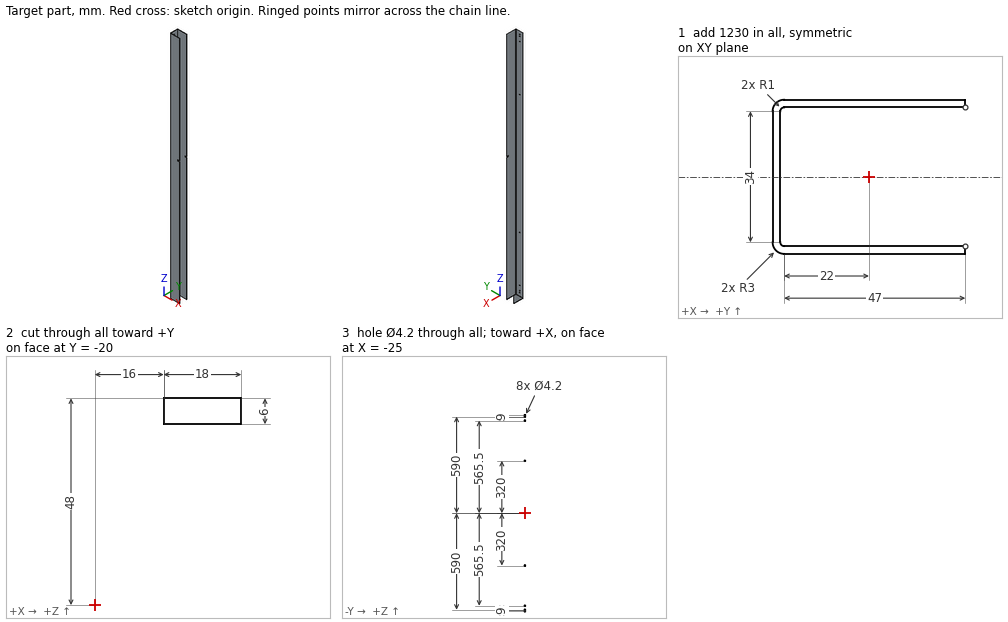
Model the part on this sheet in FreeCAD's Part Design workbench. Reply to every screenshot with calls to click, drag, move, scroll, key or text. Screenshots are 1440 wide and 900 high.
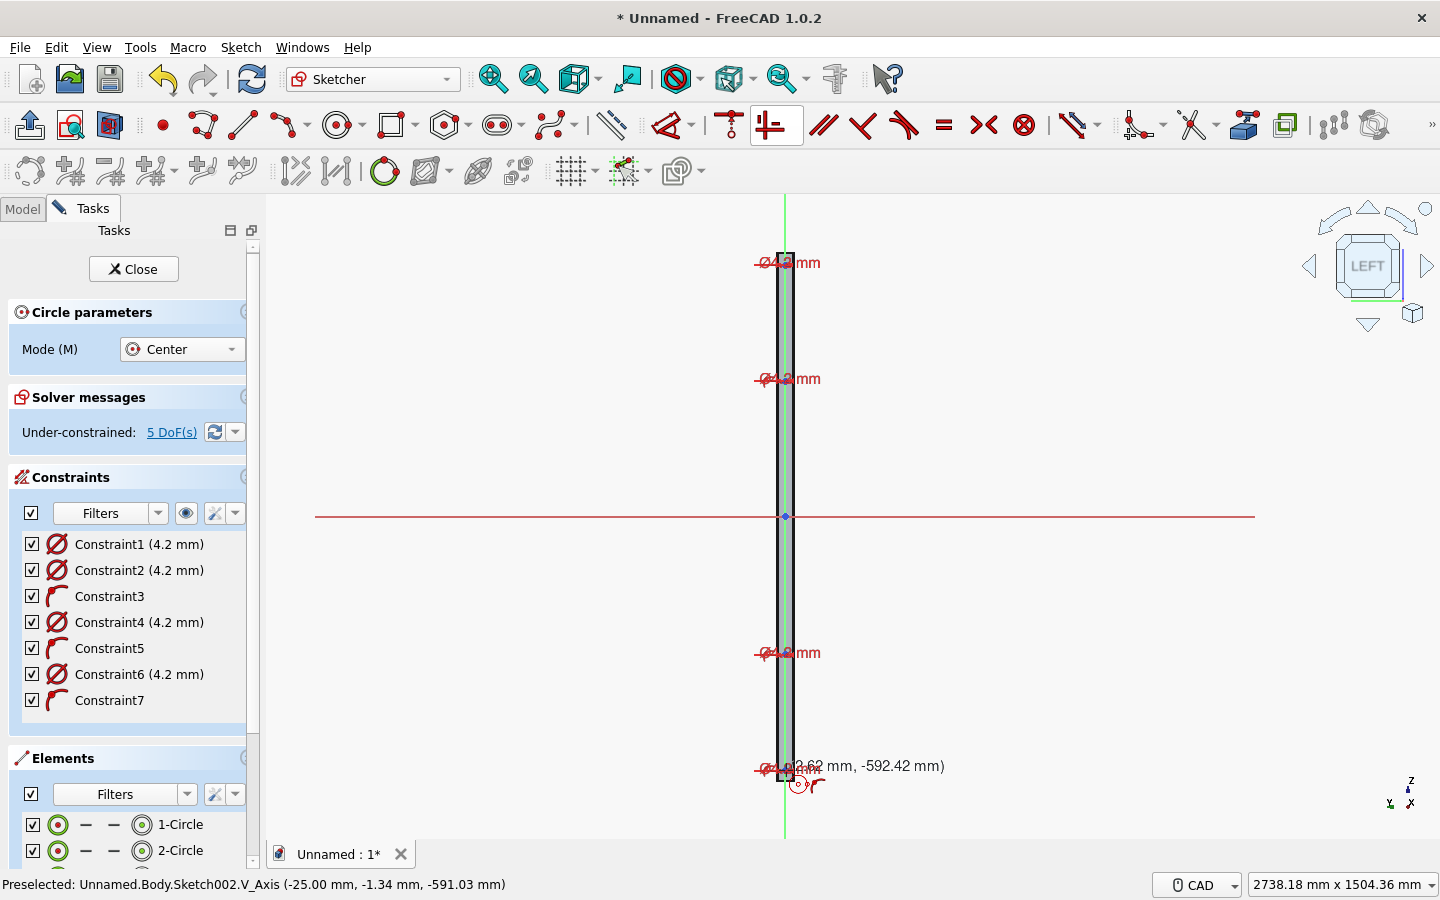
scroll(785, 274, up, 17)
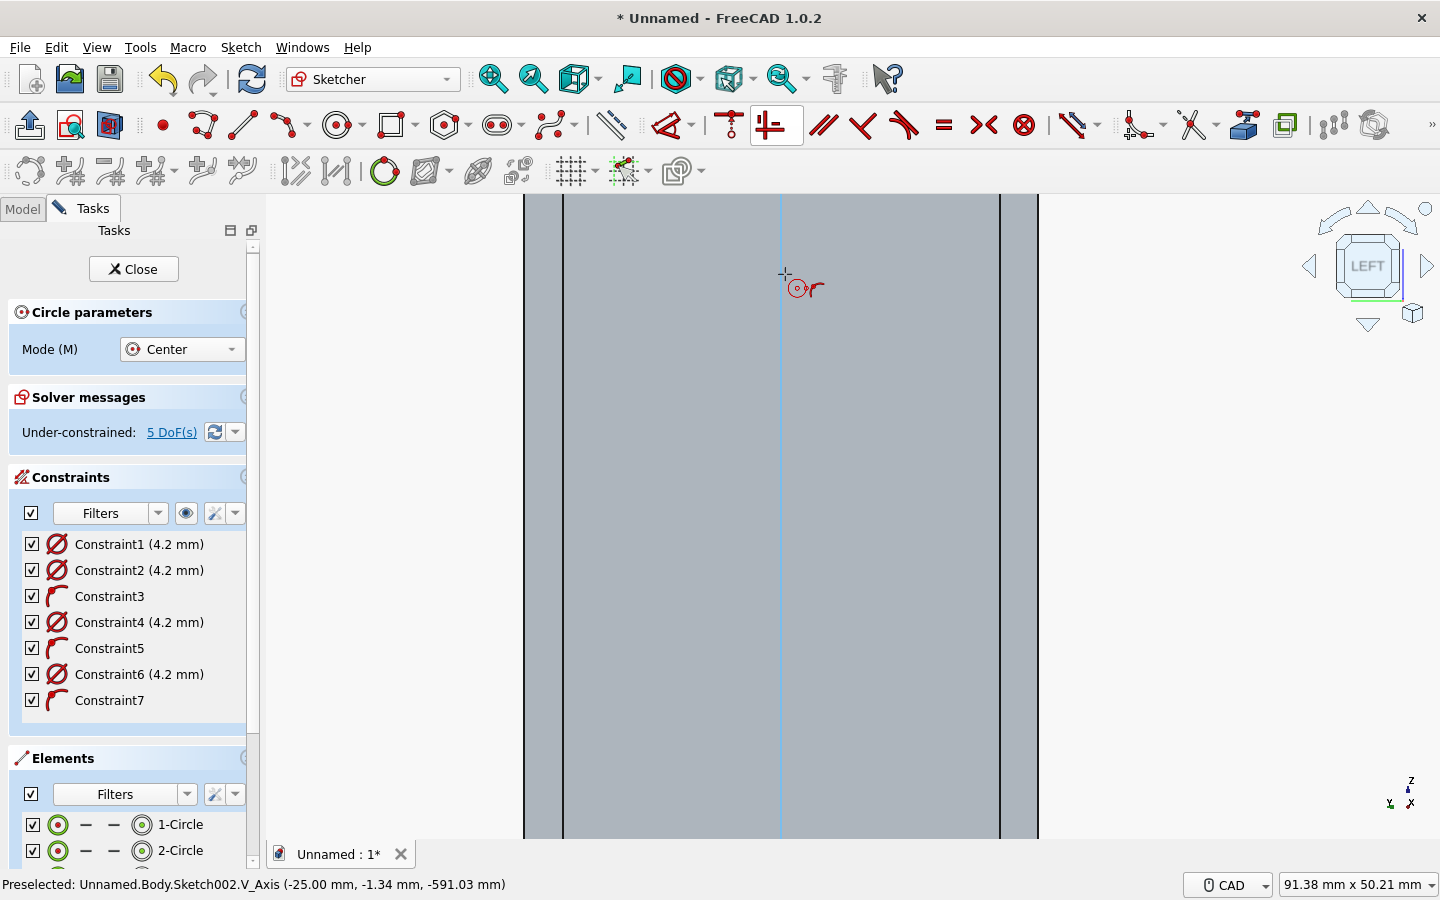
scroll(785, 274, down, 17)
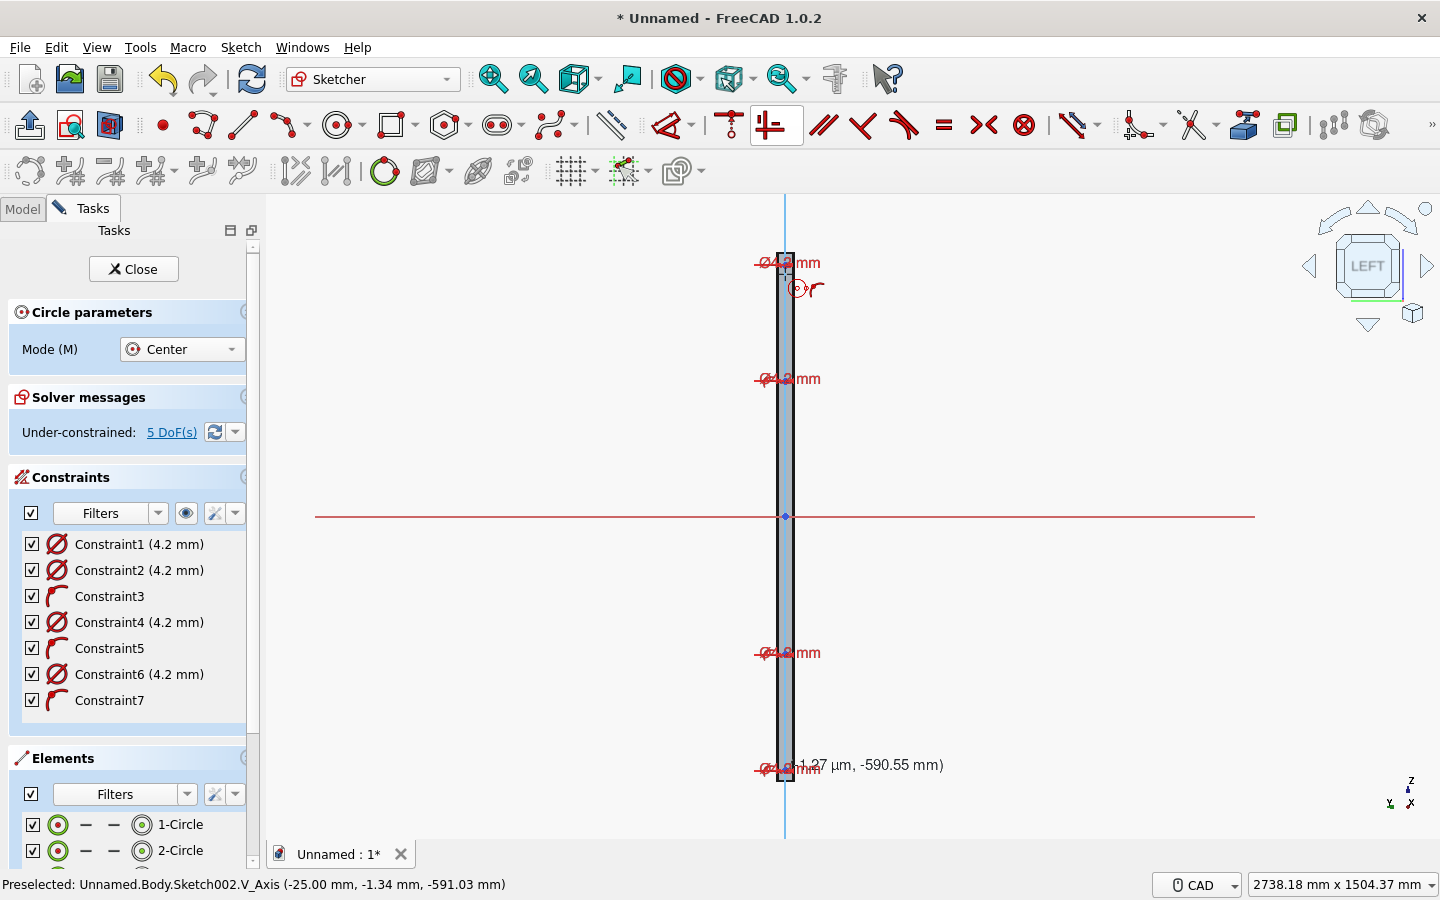
scroll(785, 274, up, 3)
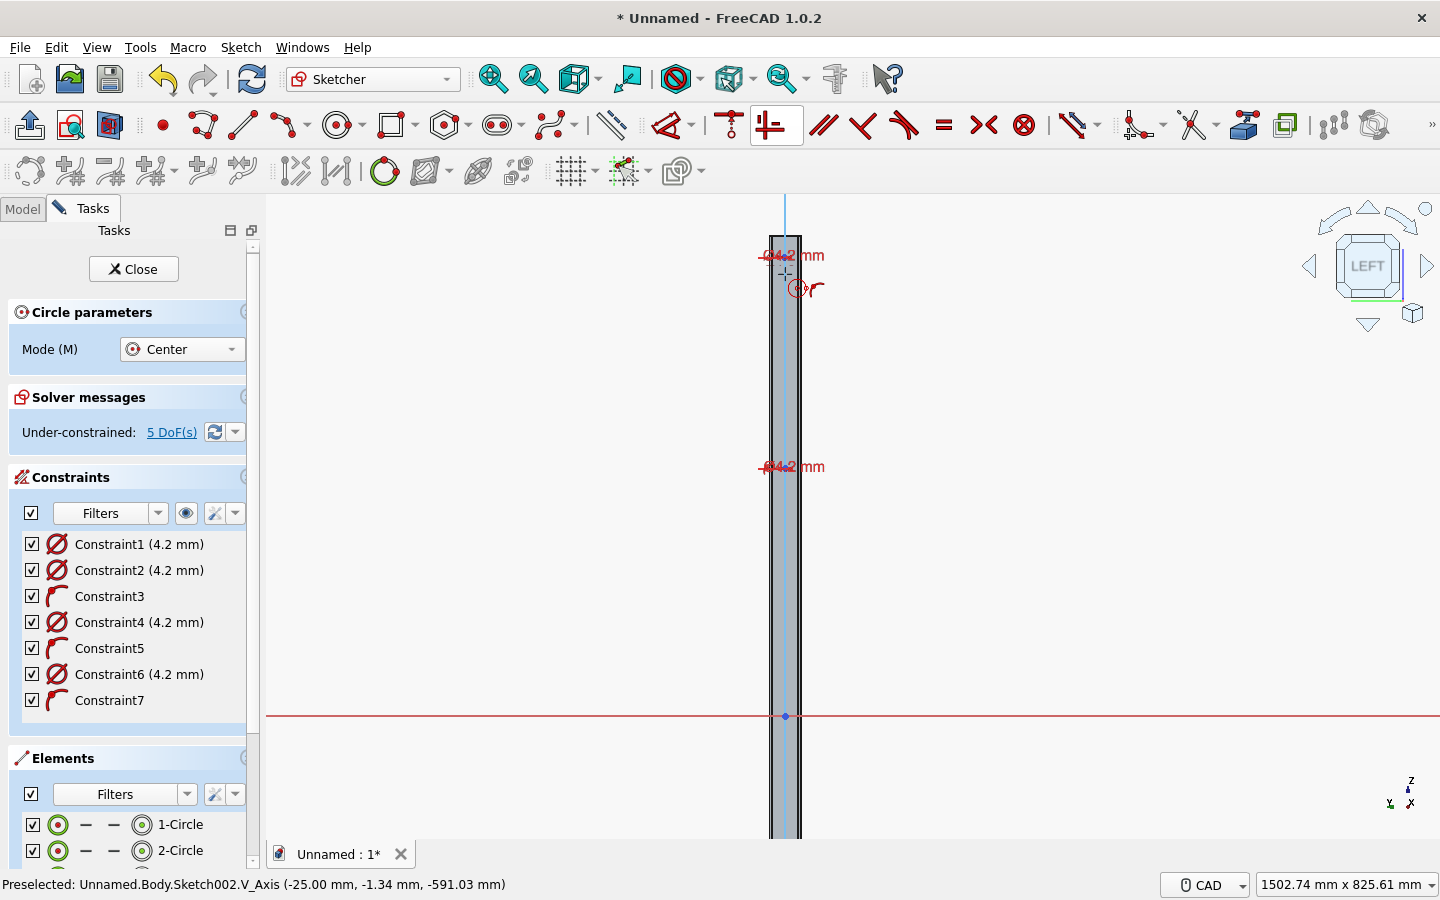
click(785, 275)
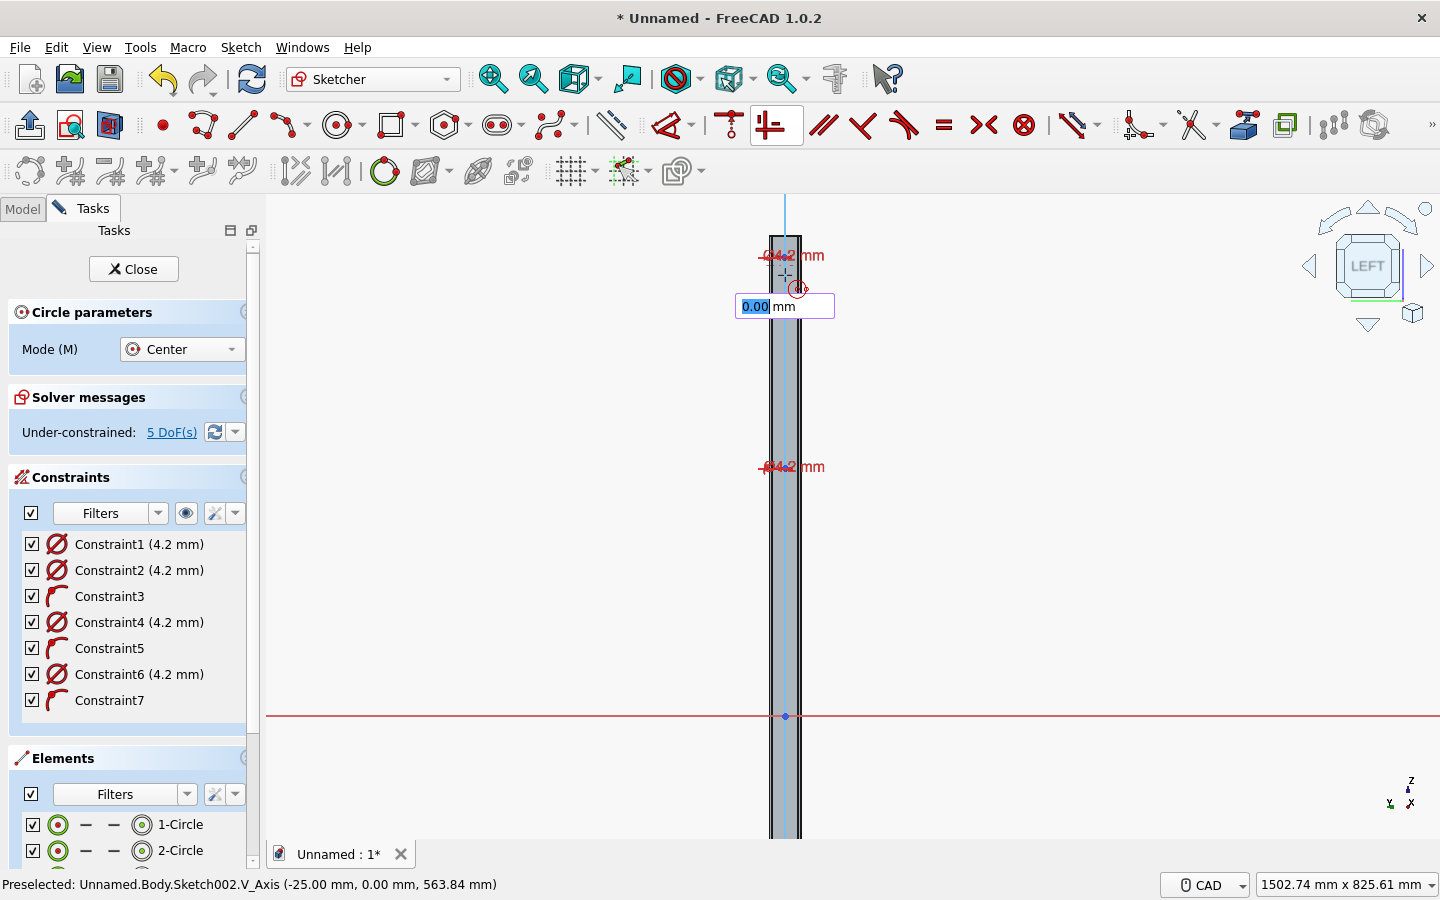
scroll(787, 274, up, 12)
move(779, 274)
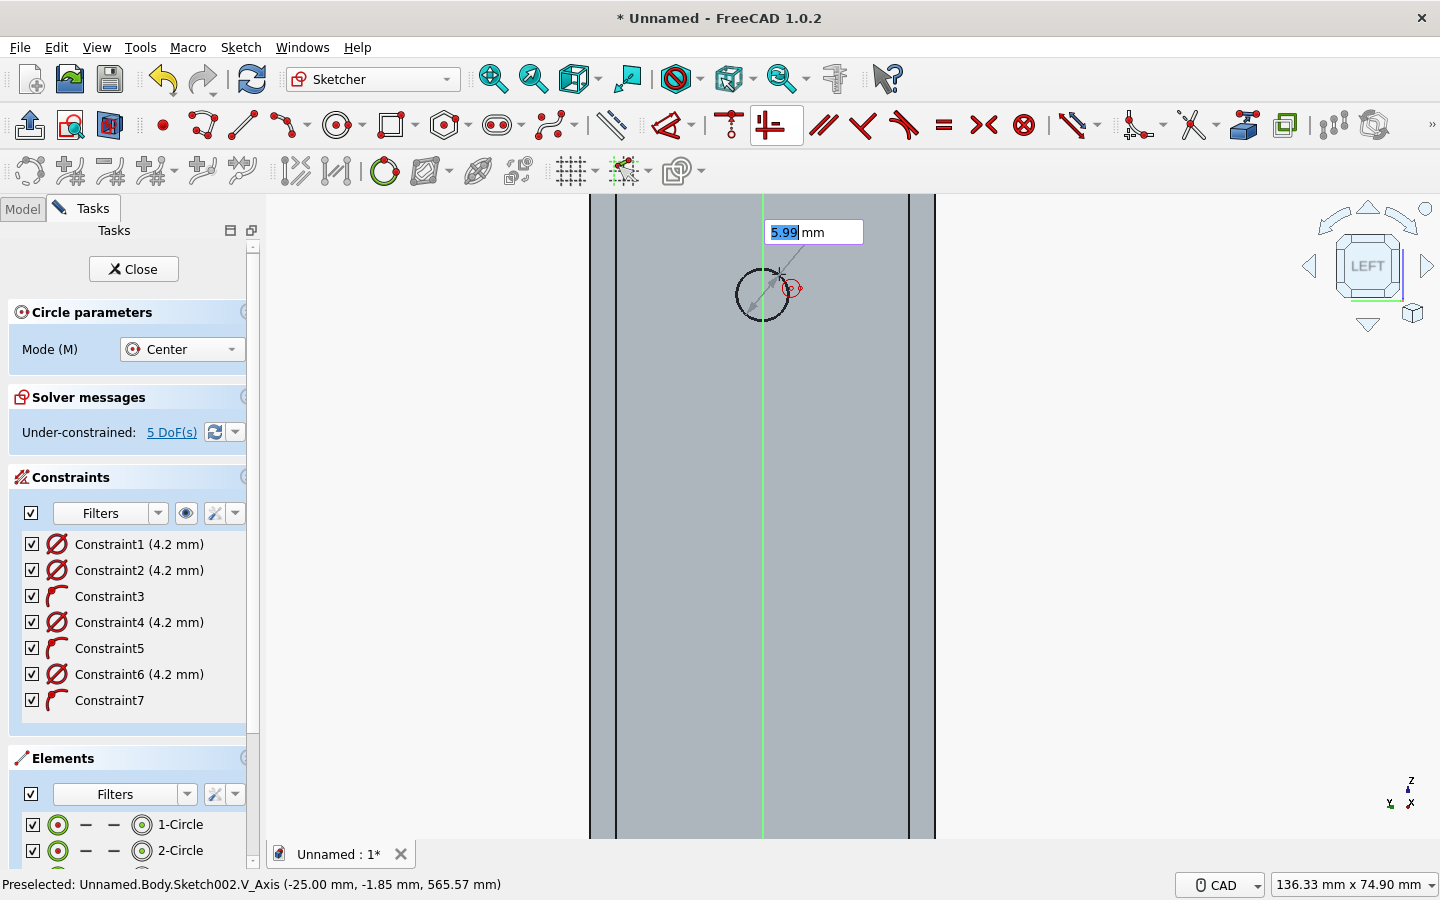
text(4.2)
key(Return)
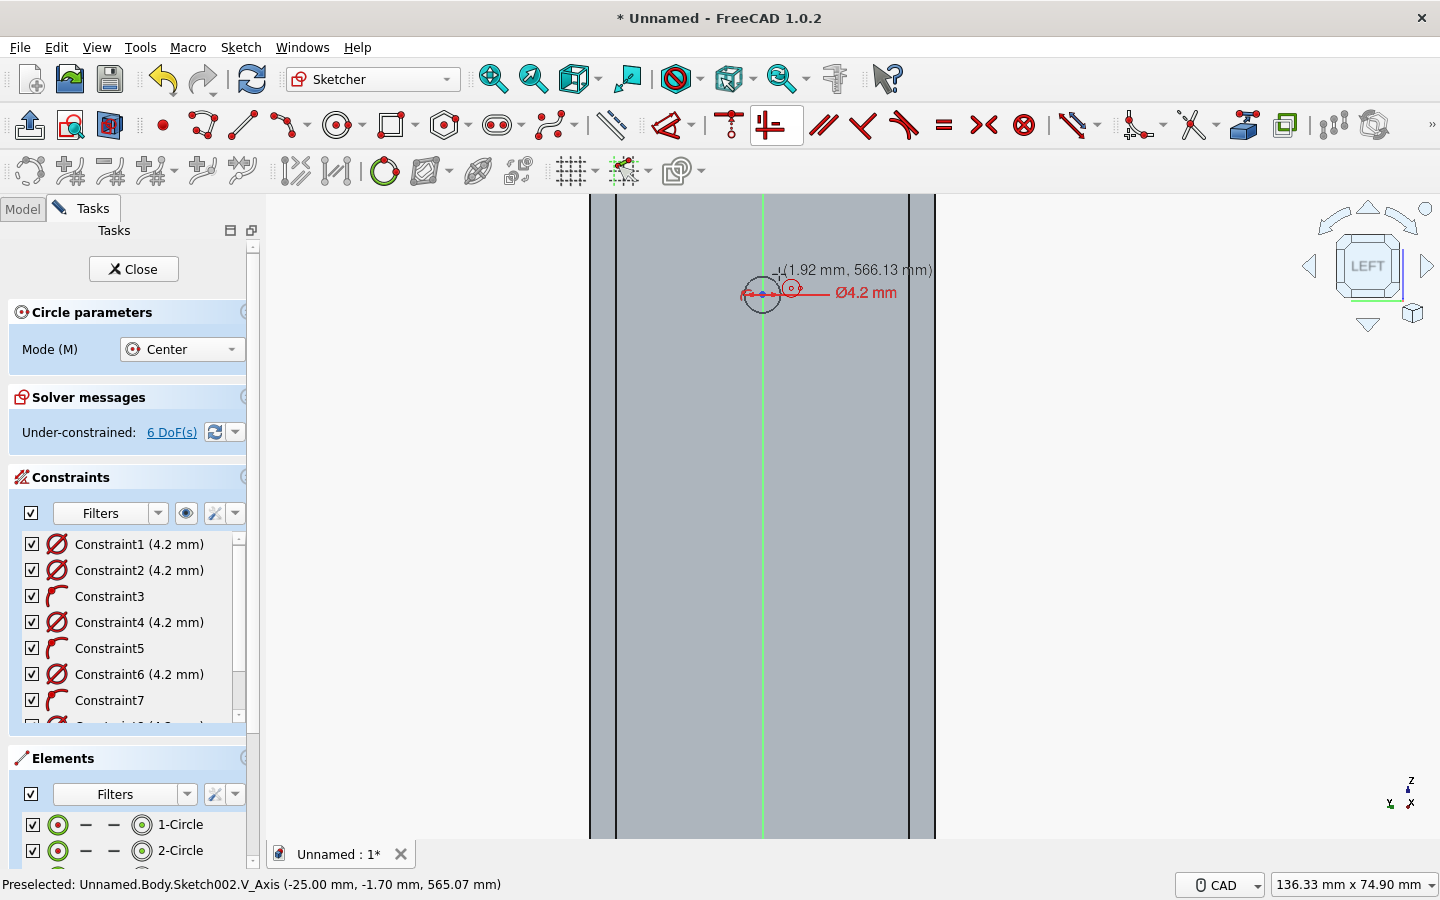
scroll(786, 274, down, 15)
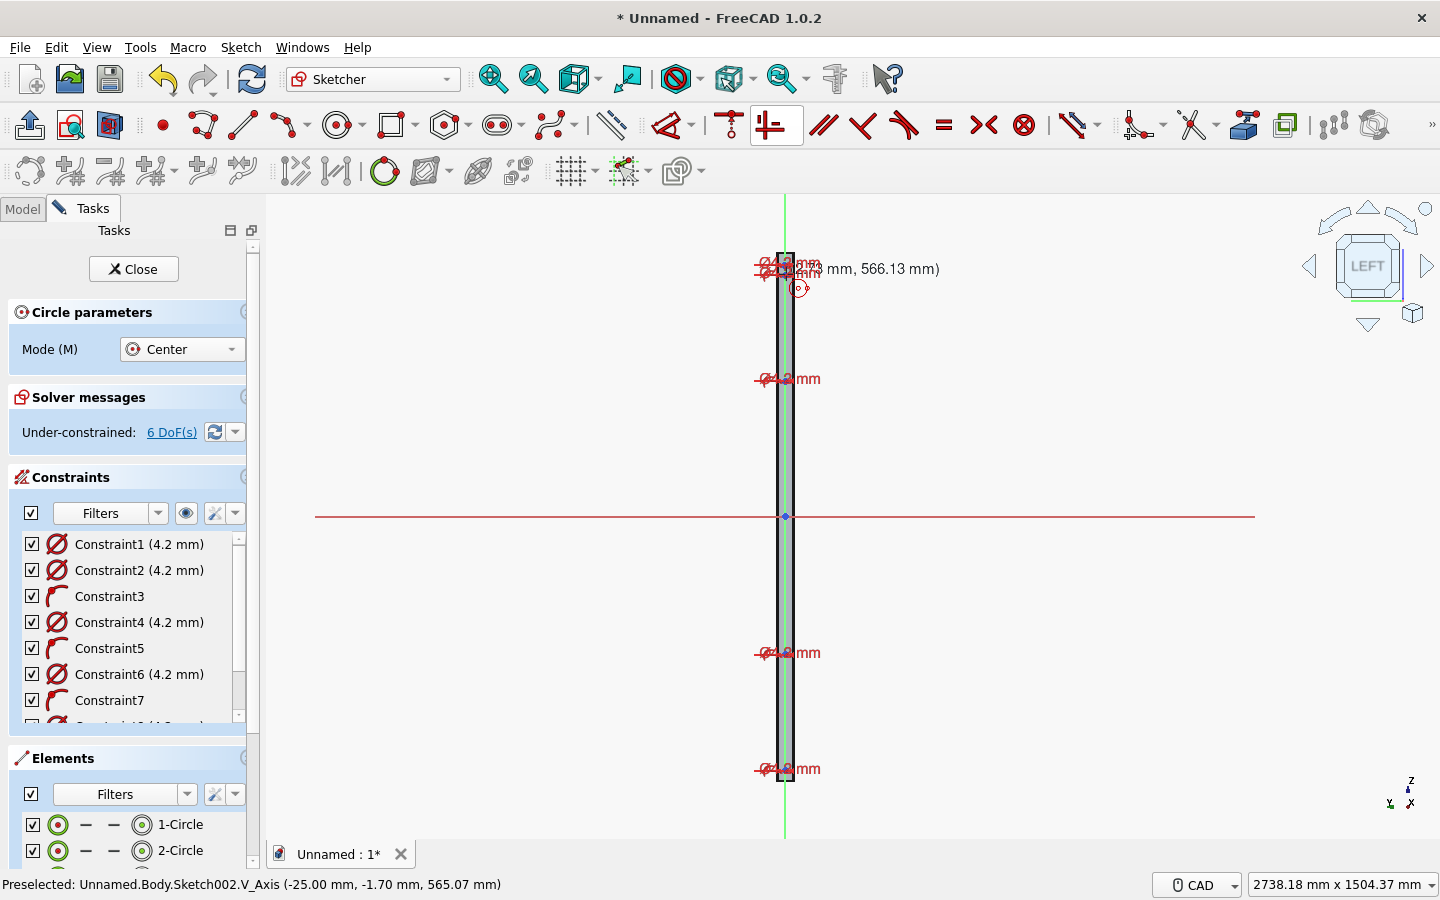
scroll(785, 260, up, 17)